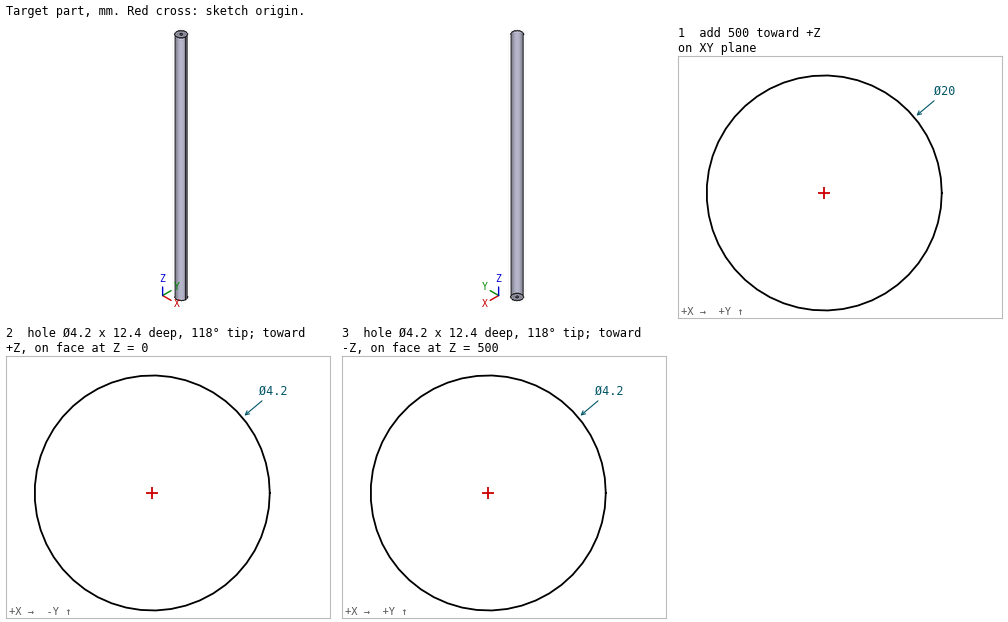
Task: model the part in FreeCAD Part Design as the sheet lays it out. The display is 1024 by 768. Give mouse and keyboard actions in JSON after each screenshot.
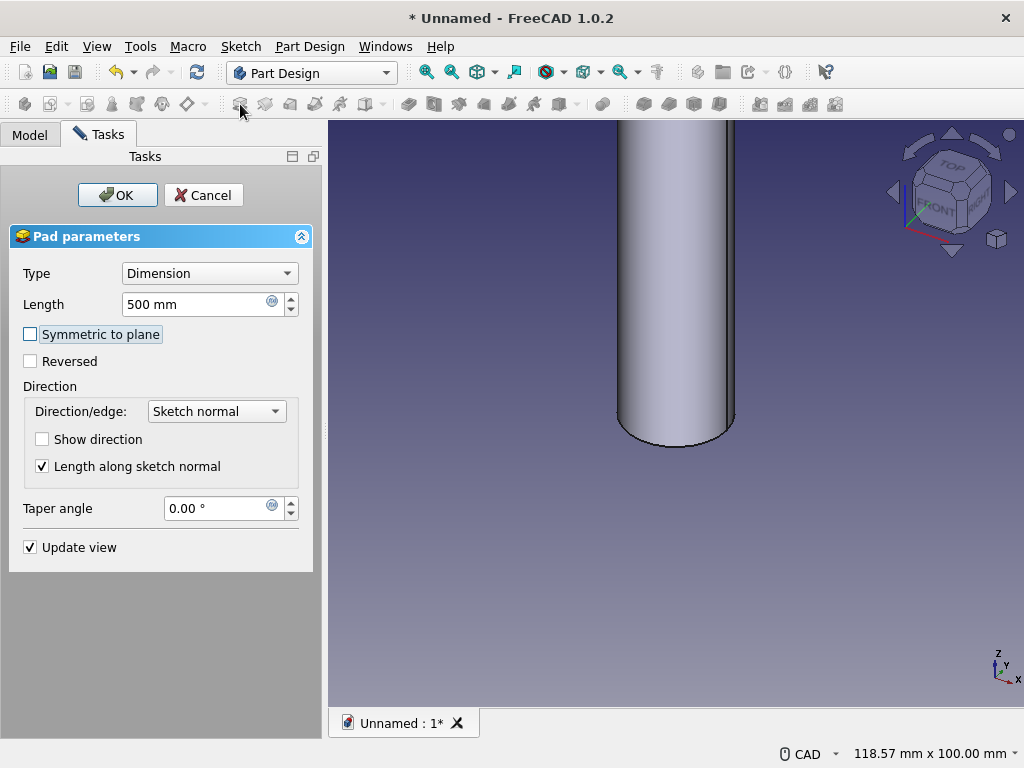
{"action": "left_click", "coordinate": [118, 195]}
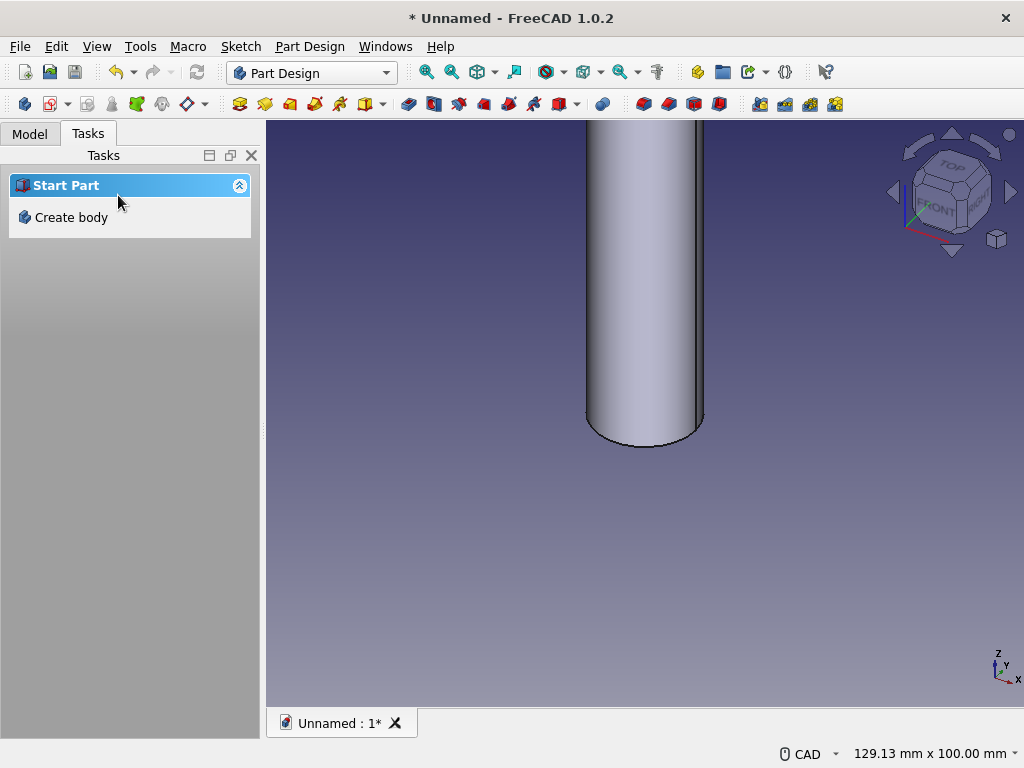
{"action": "key", "text": "v f"}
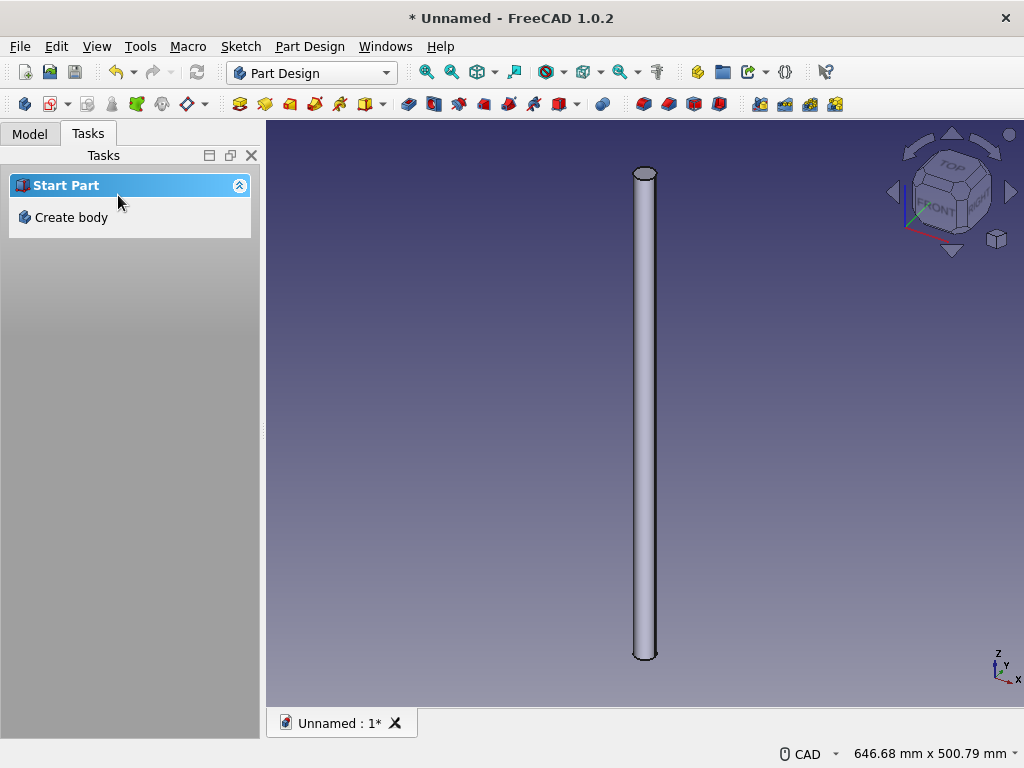
{"action": "key", "text": "5"}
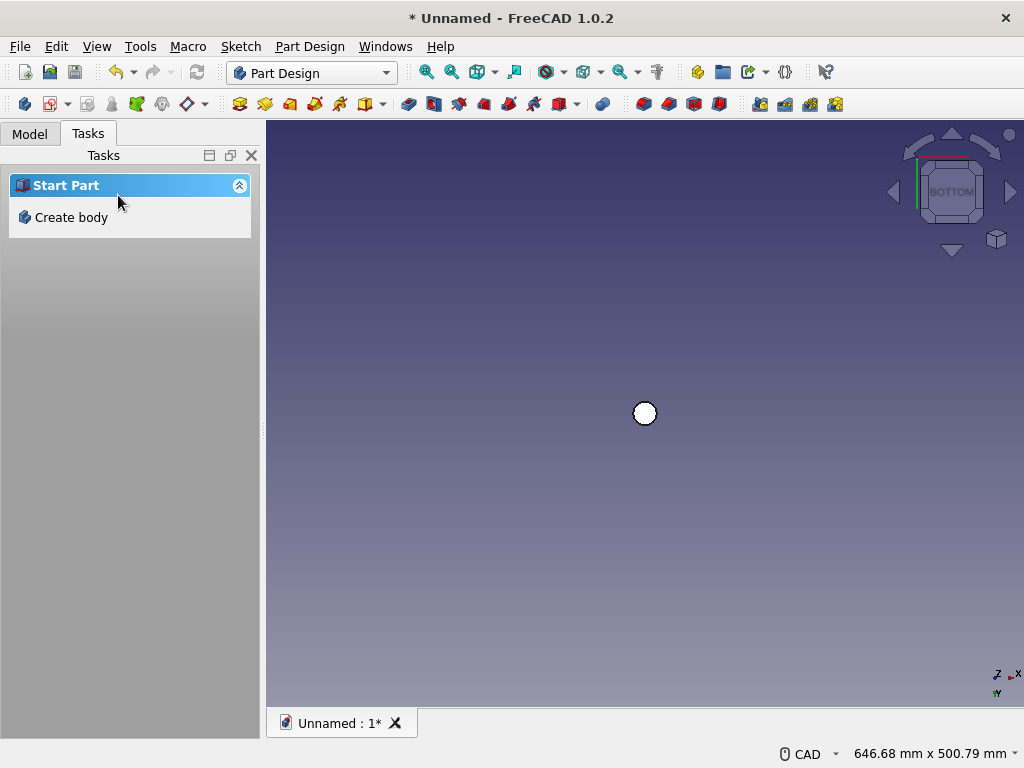
{"action": "key", "text": "v f"}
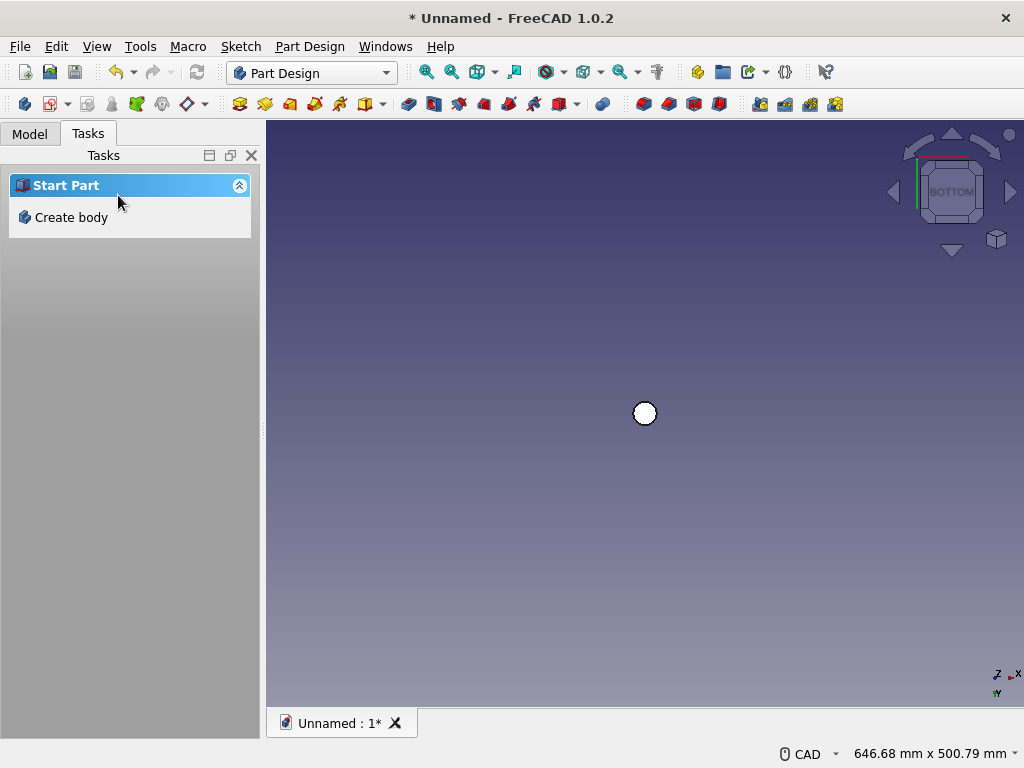
{"action": "left_click", "coordinate": [645, 412]}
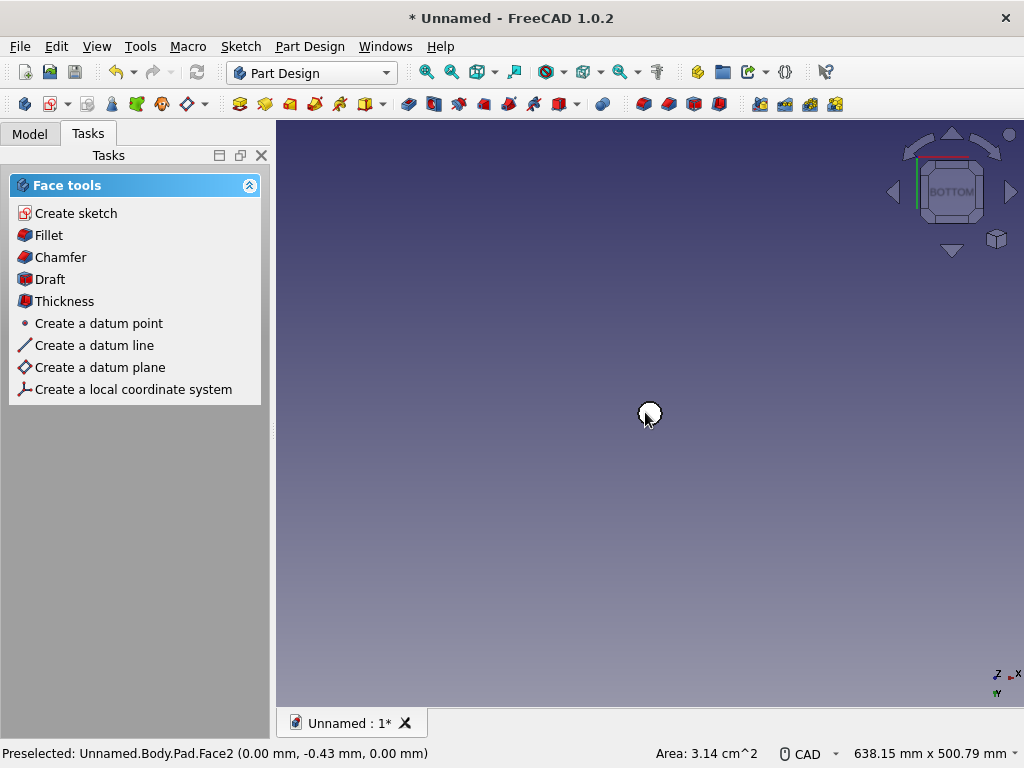
{"action": "left_click", "coordinate": [50, 104]}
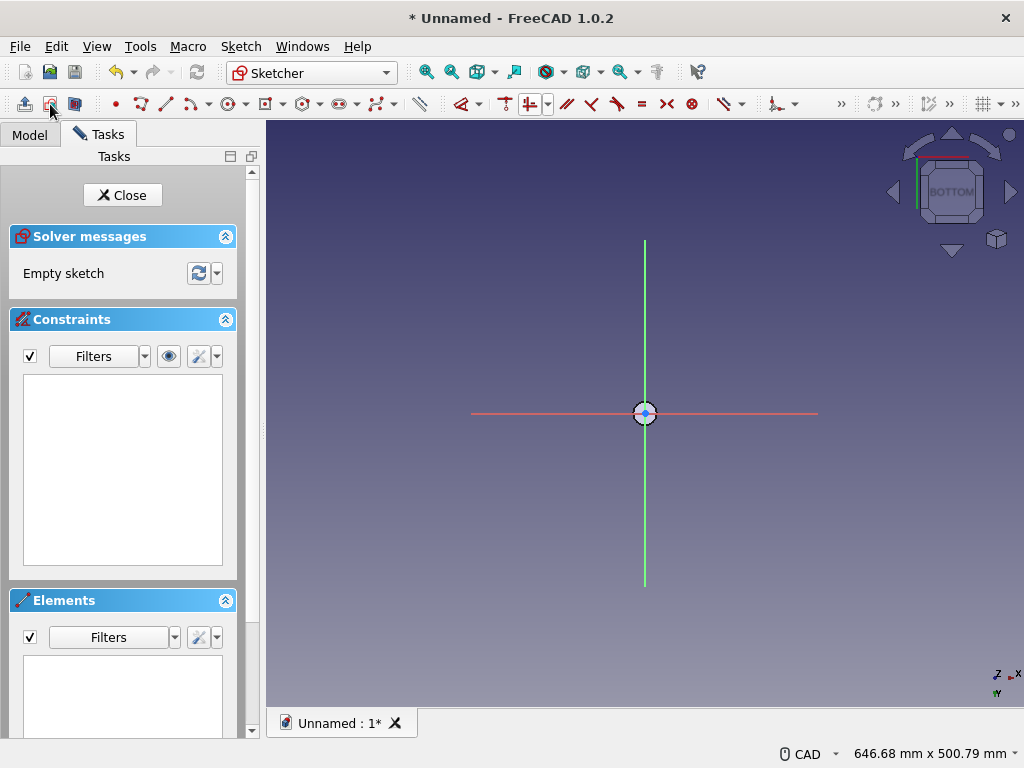
{"action": "scroll", "coordinate": [649, 414], "scroll_direction": "up", "scroll_amount": 15}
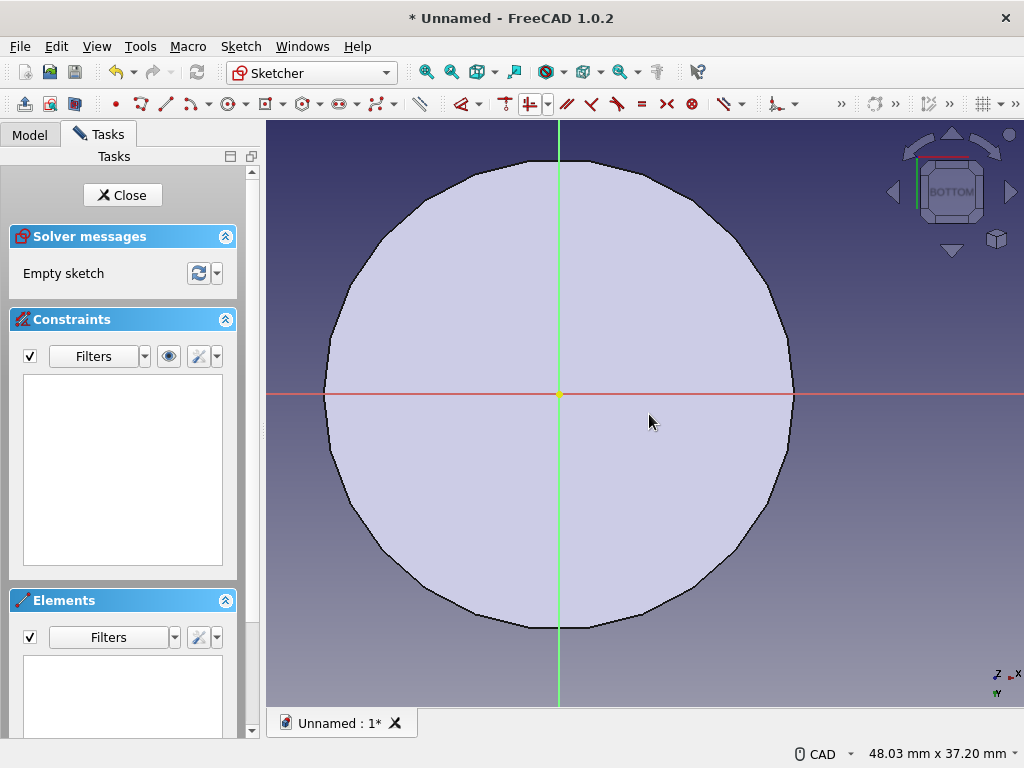
{"action": "scroll", "coordinate": [553, 388], "scroll_direction": "up", "scroll_amount": 7}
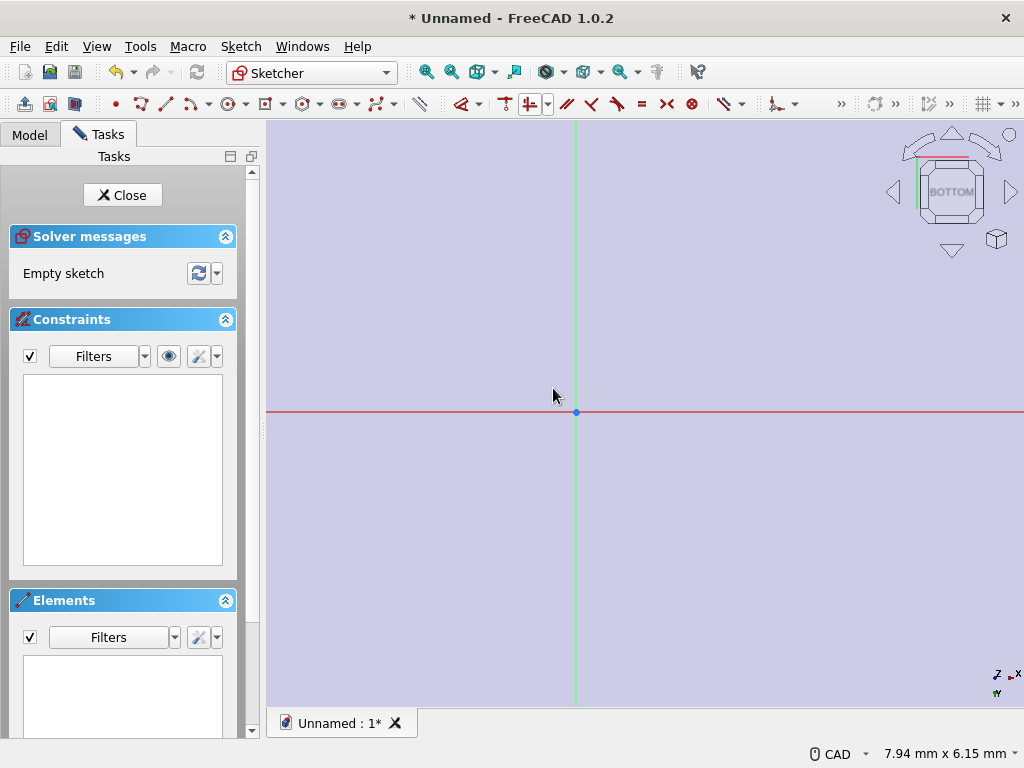
{"action": "key", "text": "g c"}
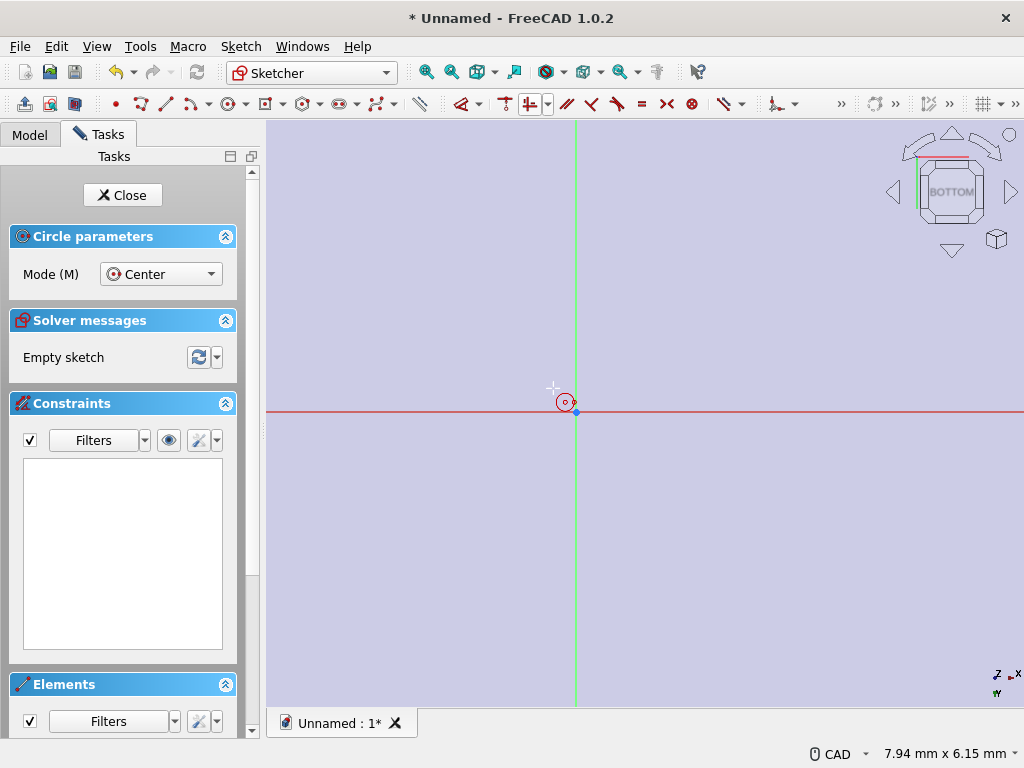
{"action": "left_click", "coordinate": [576, 412]}
{"action": "left_click", "coordinate": [718, 271]}
{"action": "key", "text": "Escape"}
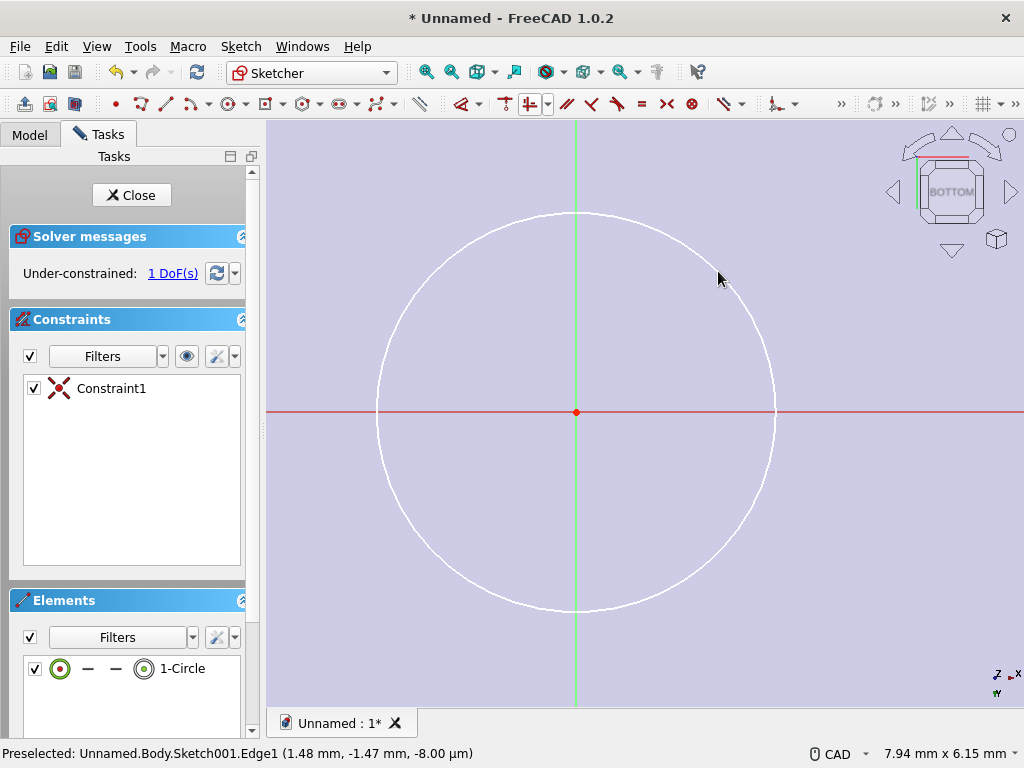
{"action": "left_click", "coordinate": [717, 271]}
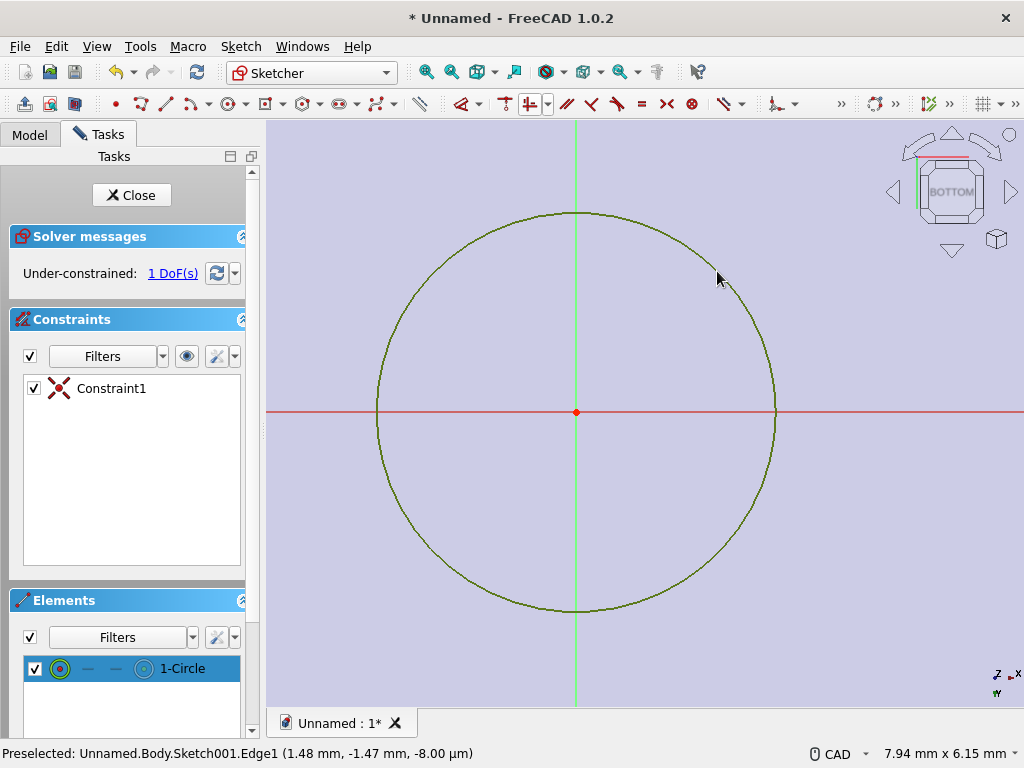
{"action": "key", "text": "k o"}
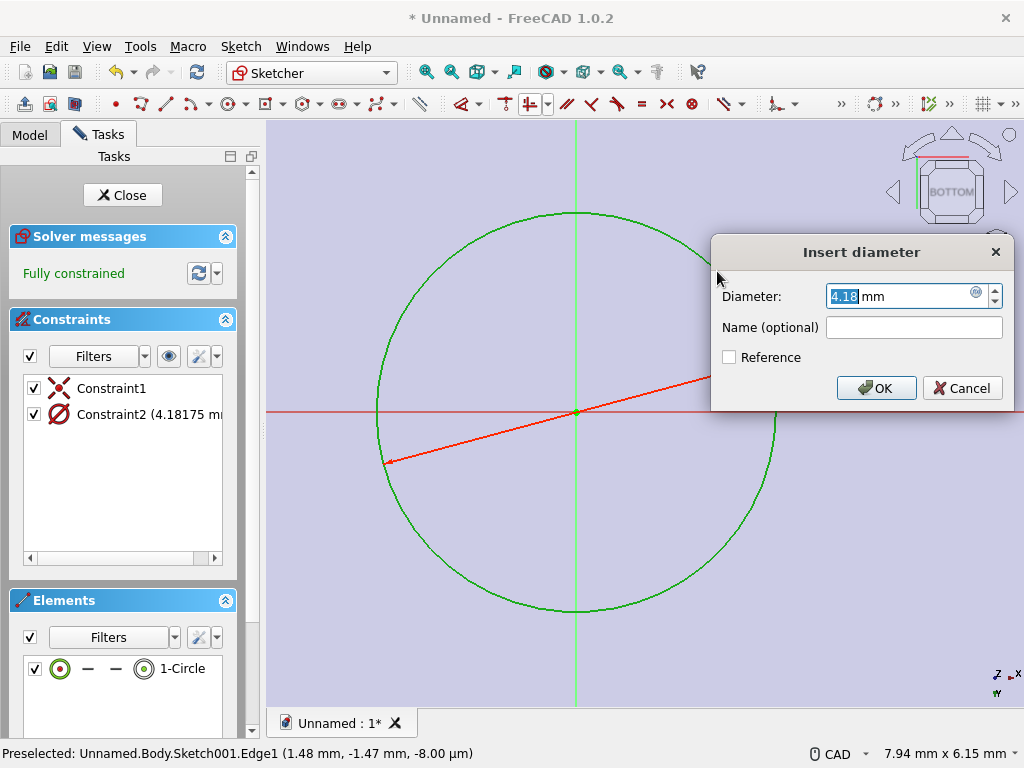
{"action": "type", "text": "4.2"}
{"action": "key", "text": "Return"}